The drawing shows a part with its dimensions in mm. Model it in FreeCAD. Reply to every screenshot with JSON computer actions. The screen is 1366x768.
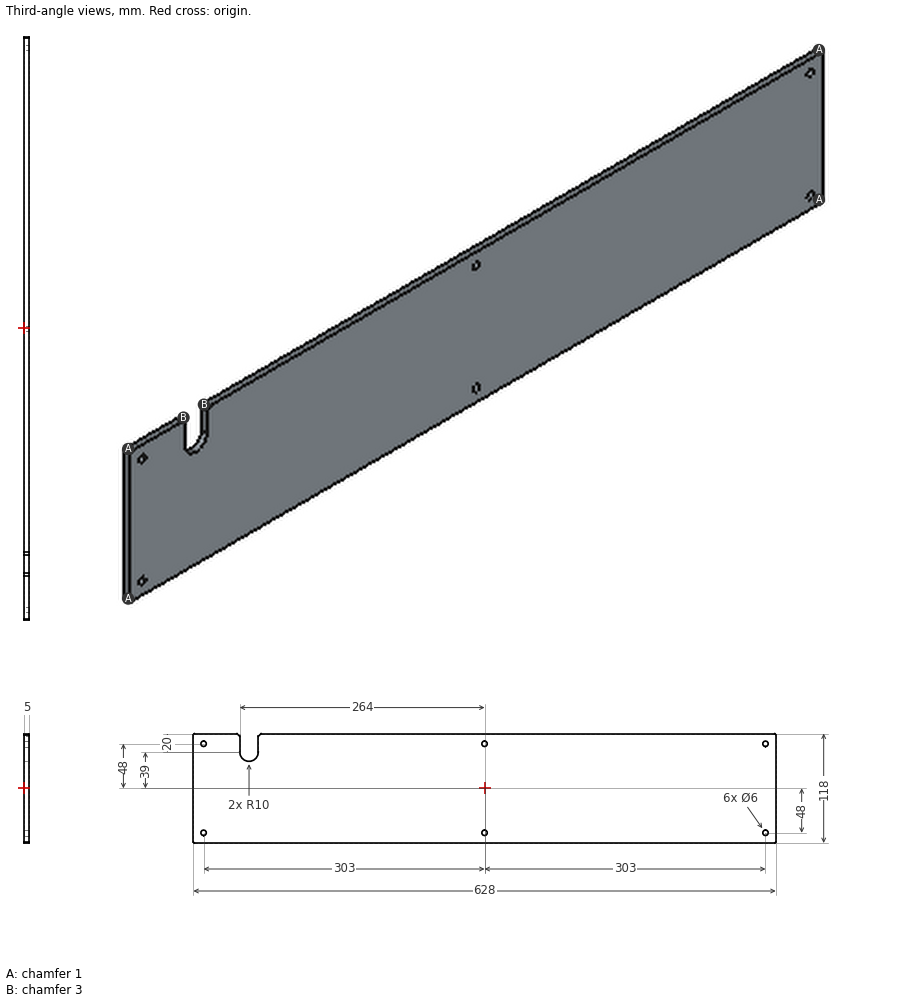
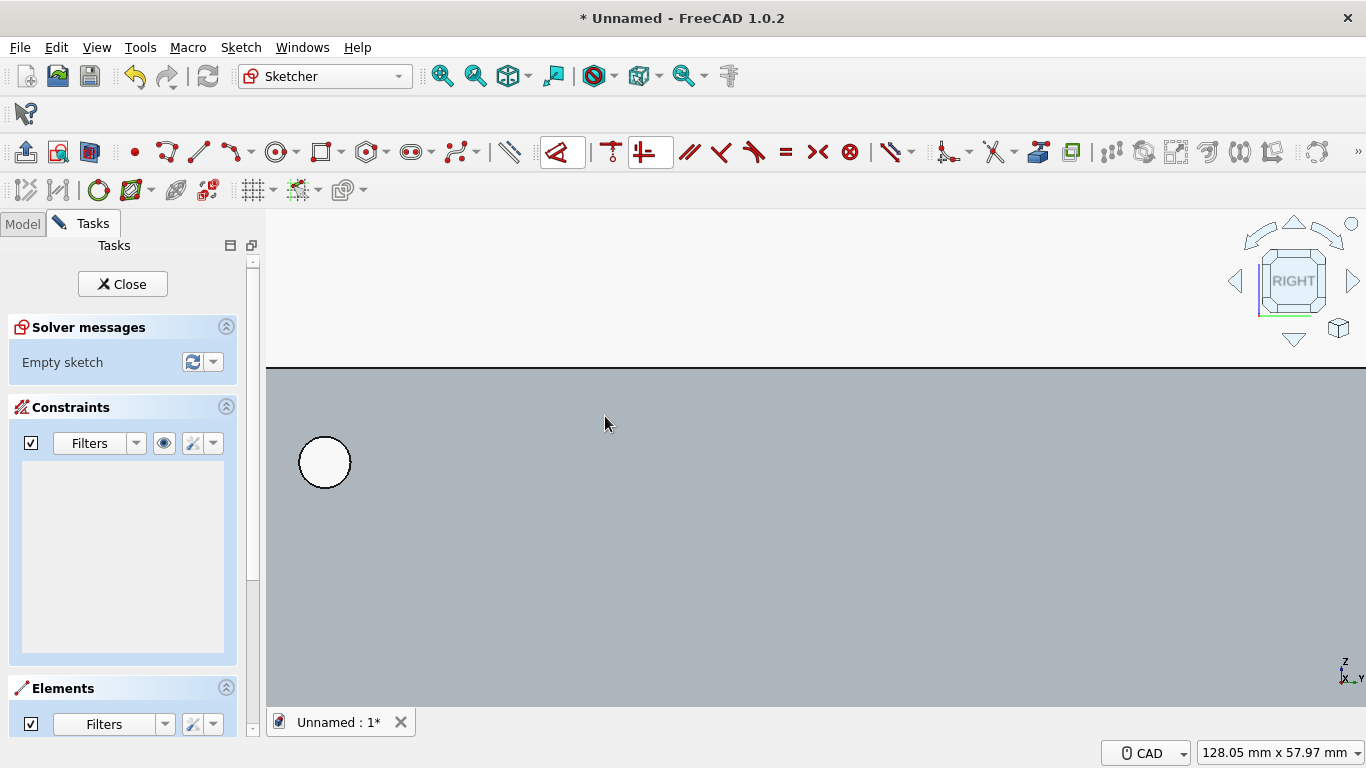
{"action": "left_click", "coordinate": [412, 152]}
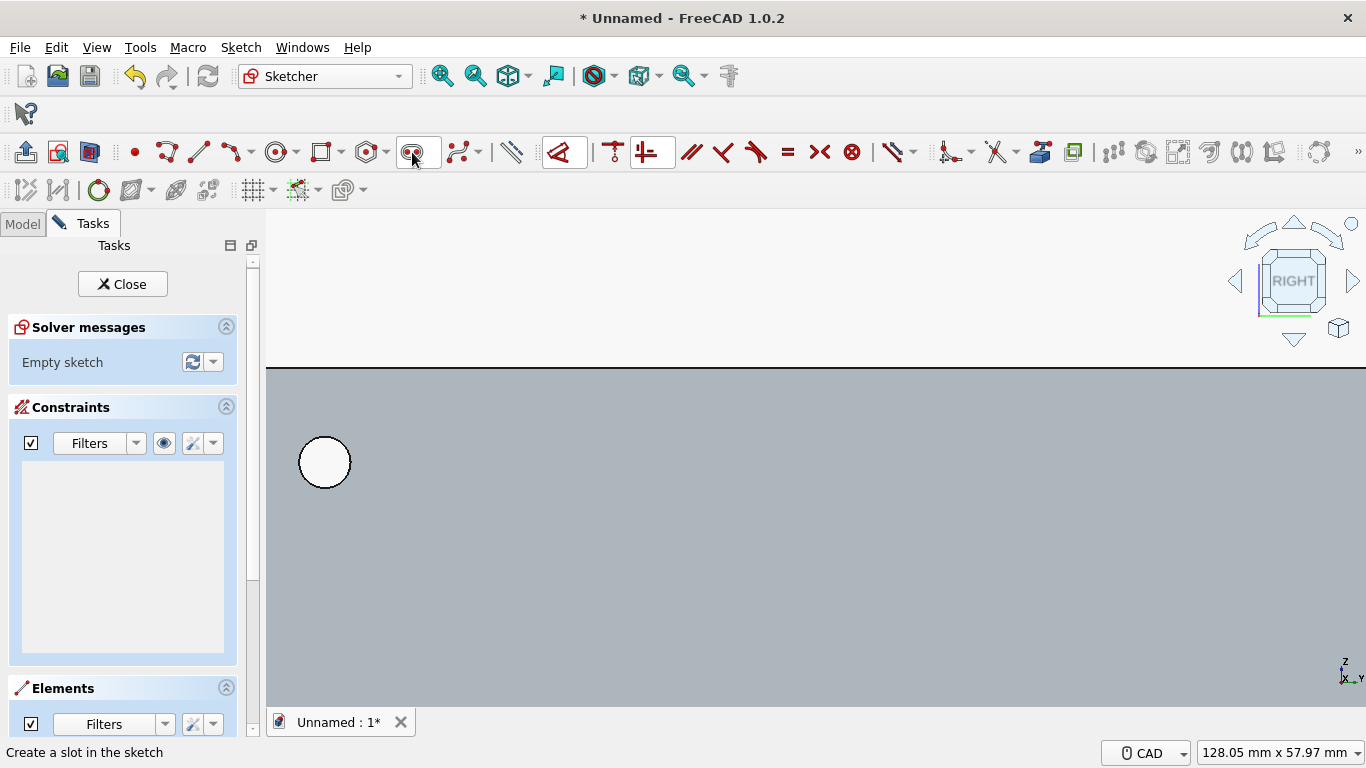
{"action": "left_click", "coordinate": [746, 540]}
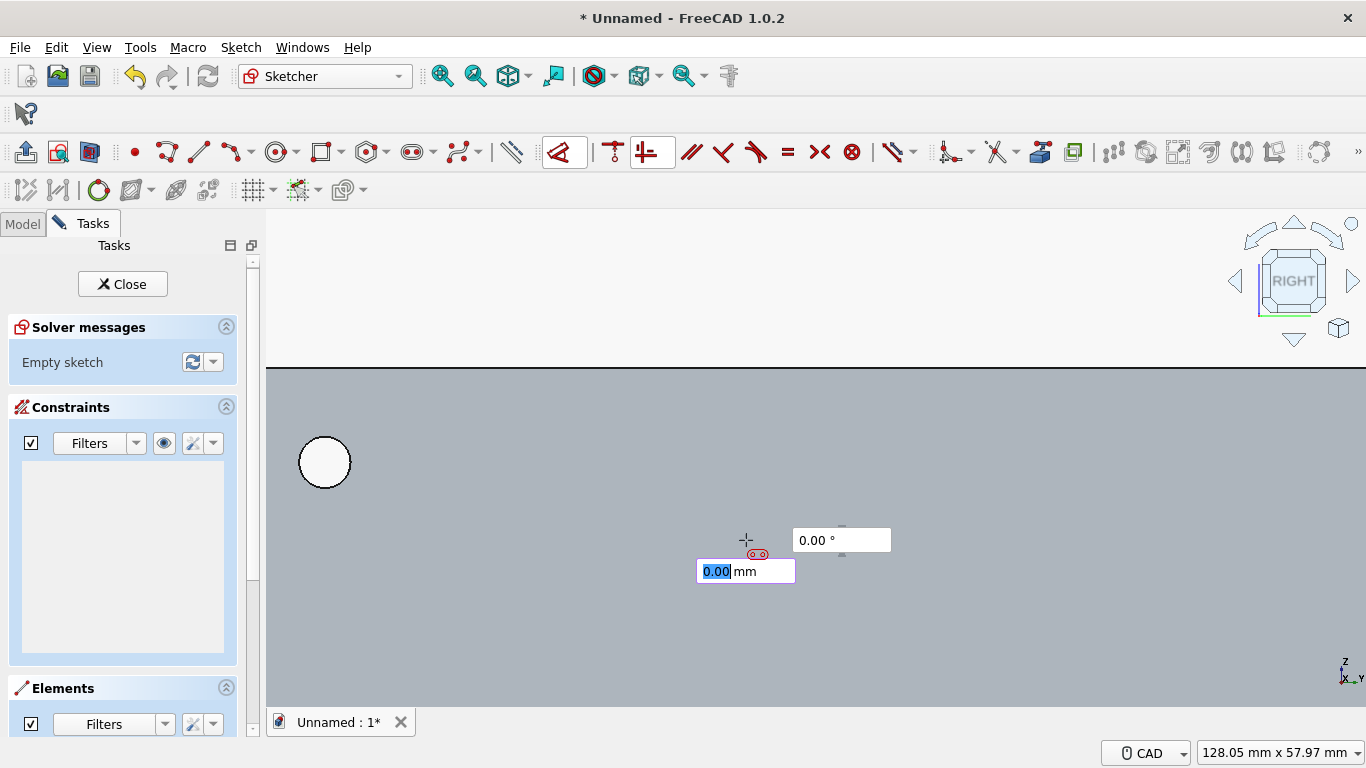
{"action": "left_click", "coordinate": [746, 368]}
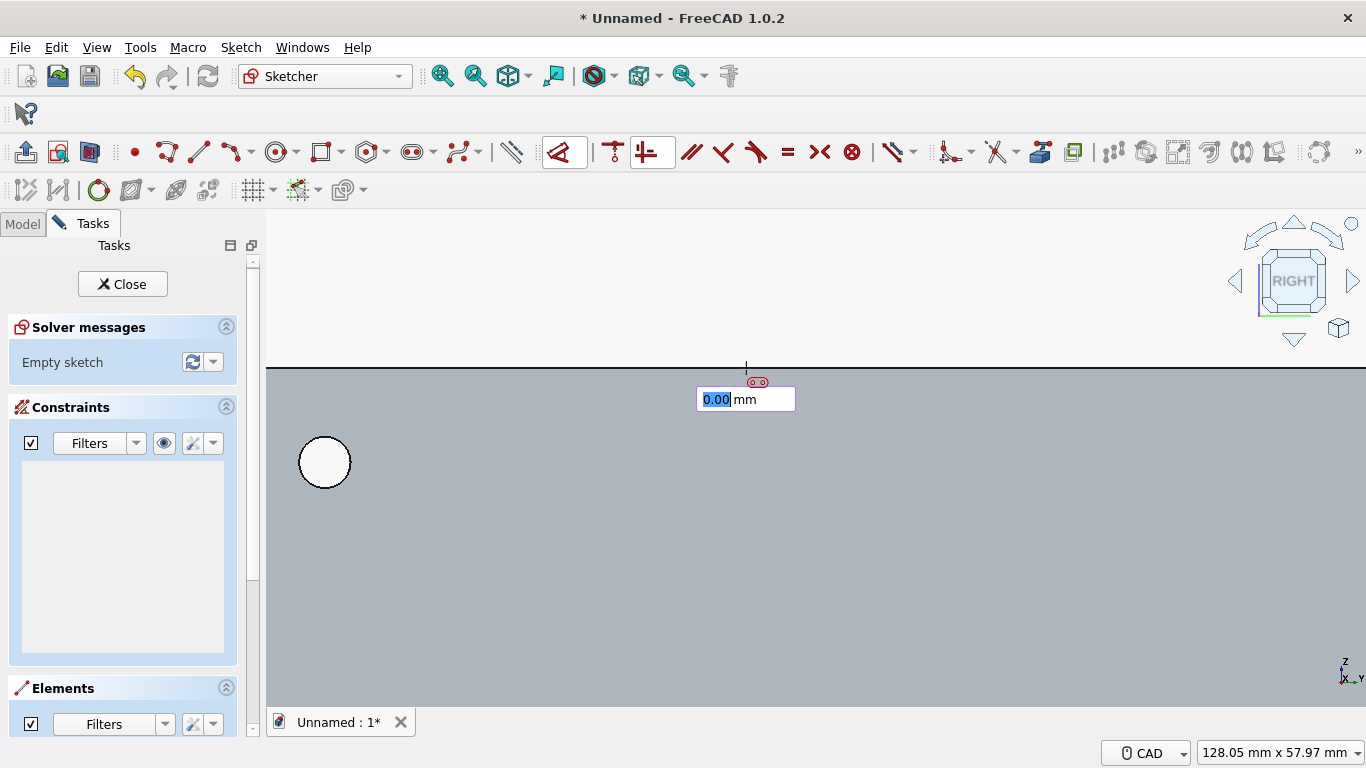
{"action": "left_click", "coordinate": [660, 454]}
{"action": "key", "text": "Escape"}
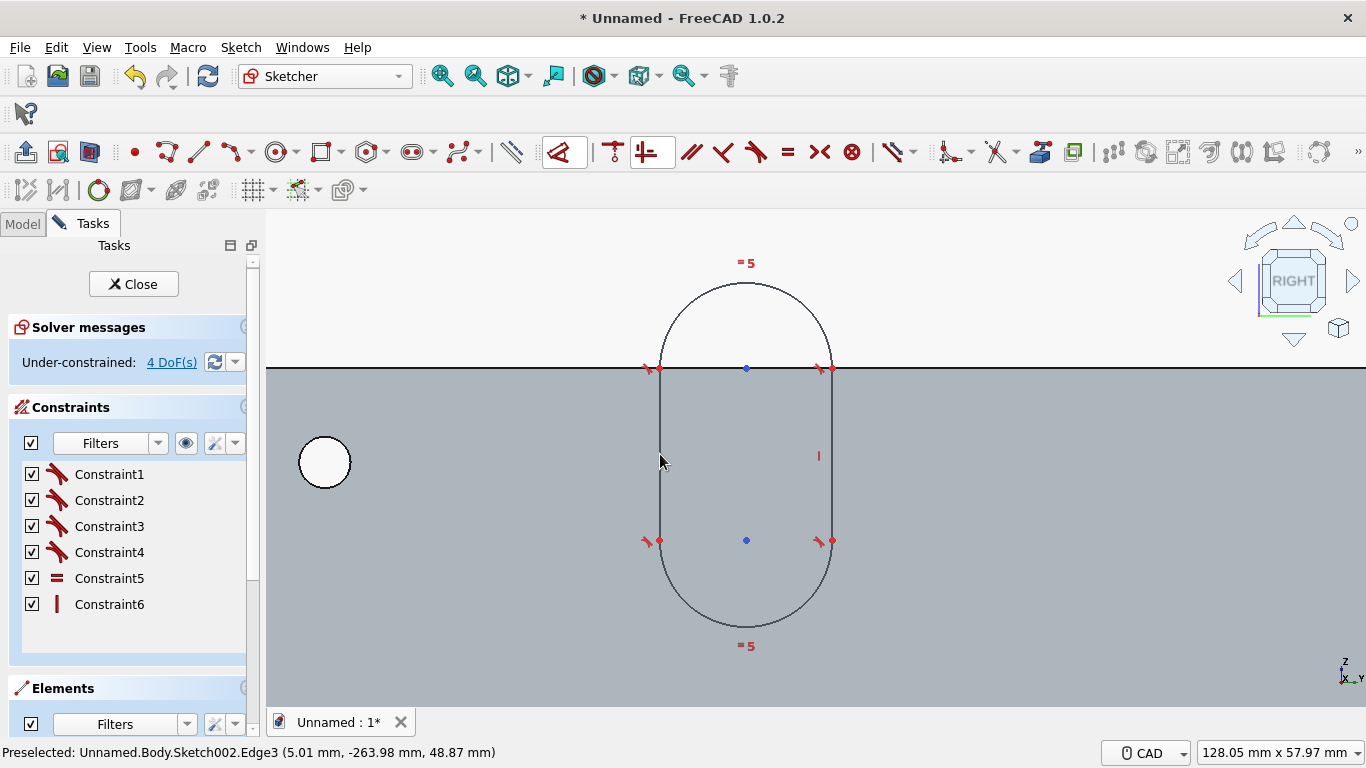
{"action": "left_click", "coordinate": [695, 611]}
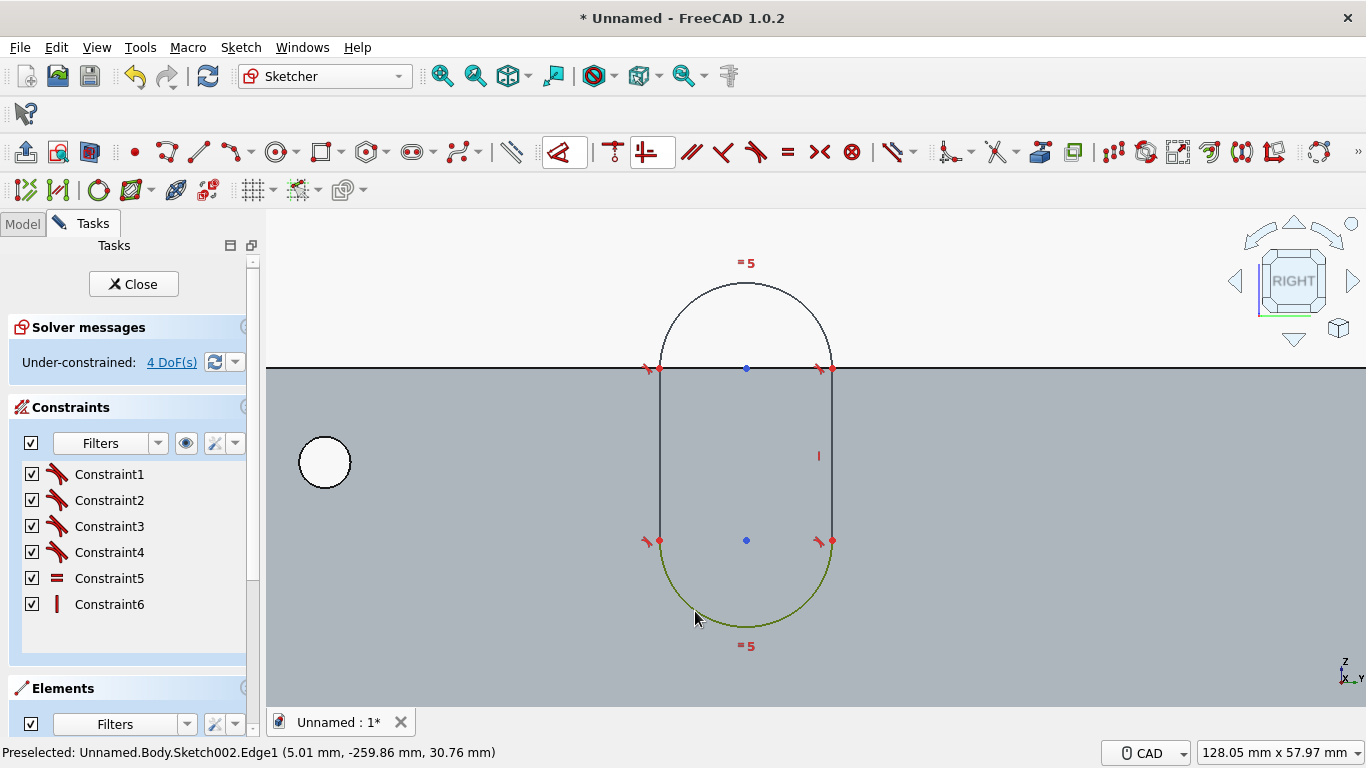
{"action": "key", "text": "k r"}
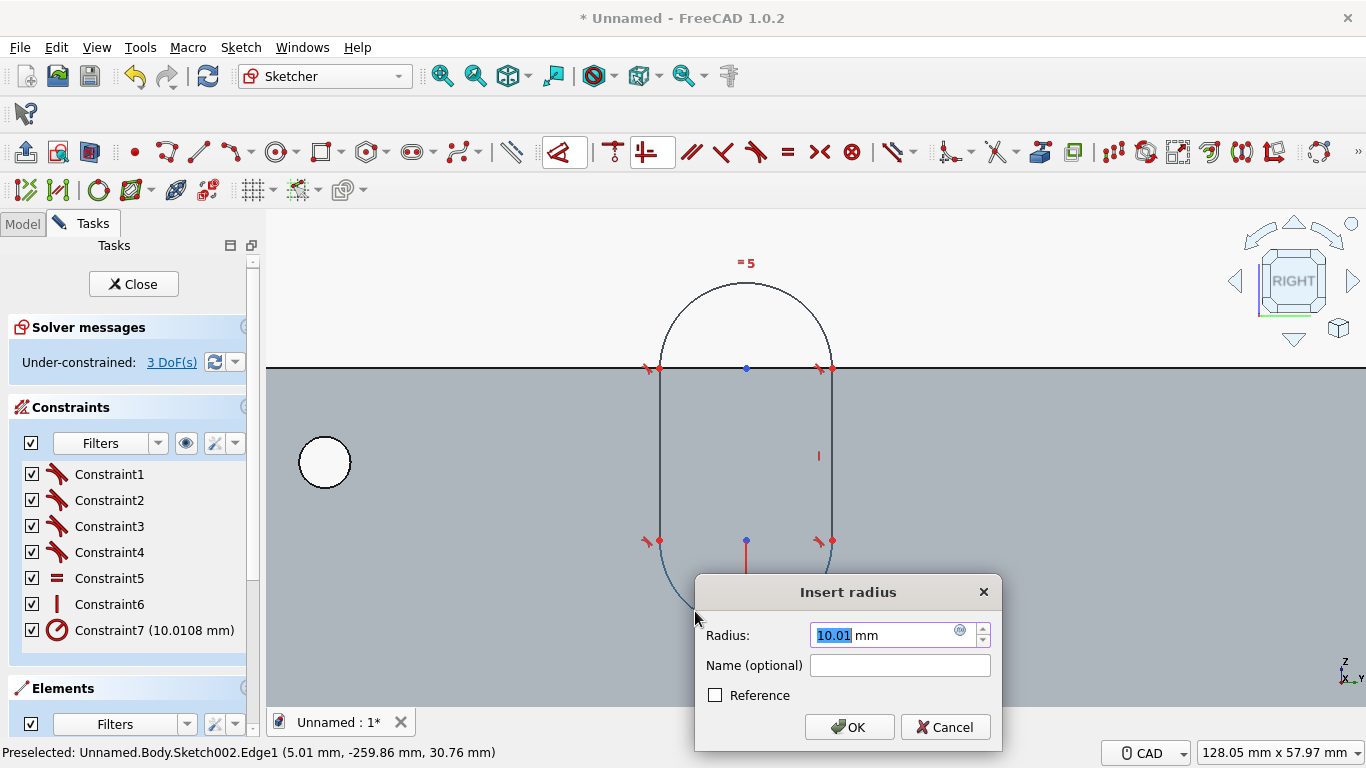
{"action": "type", "text": "10"}
{"action": "key", "text": "Return"}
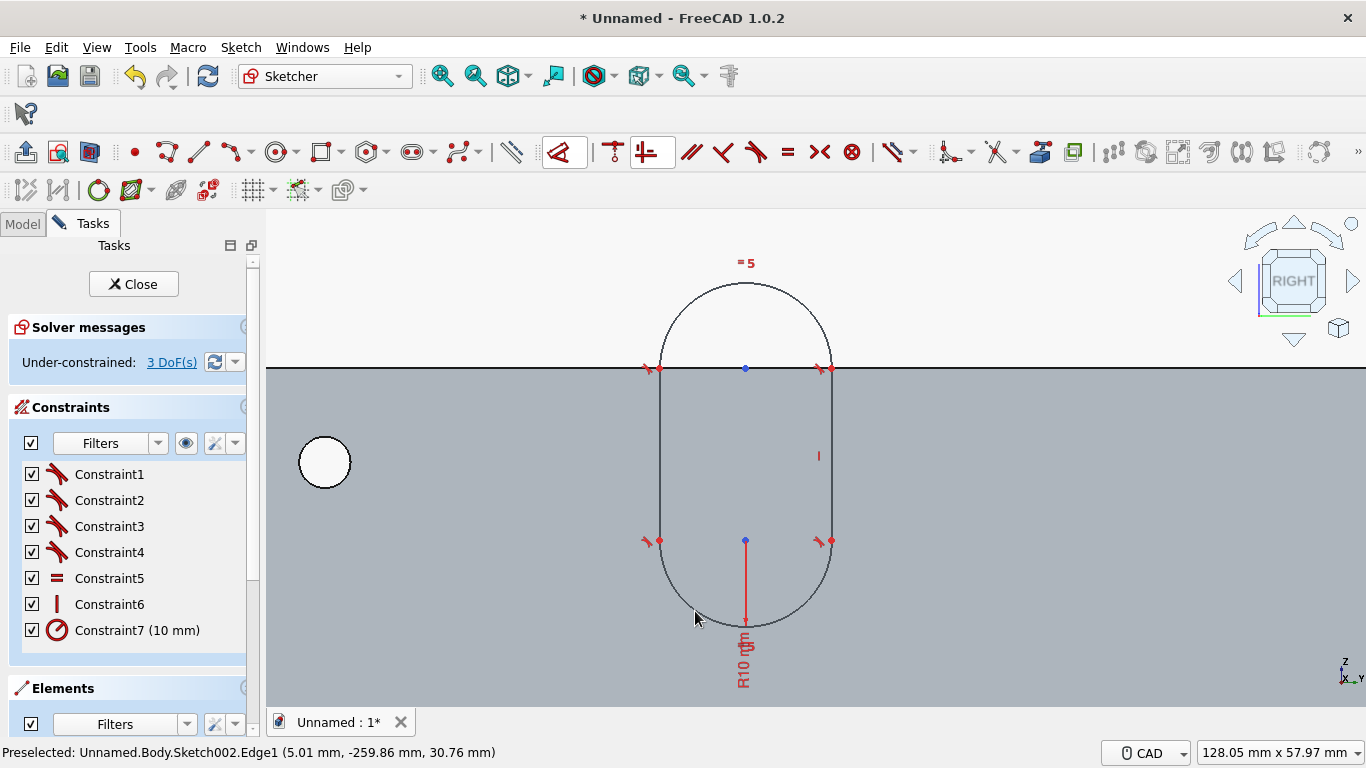
{"action": "left_click", "coordinate": [660, 489]}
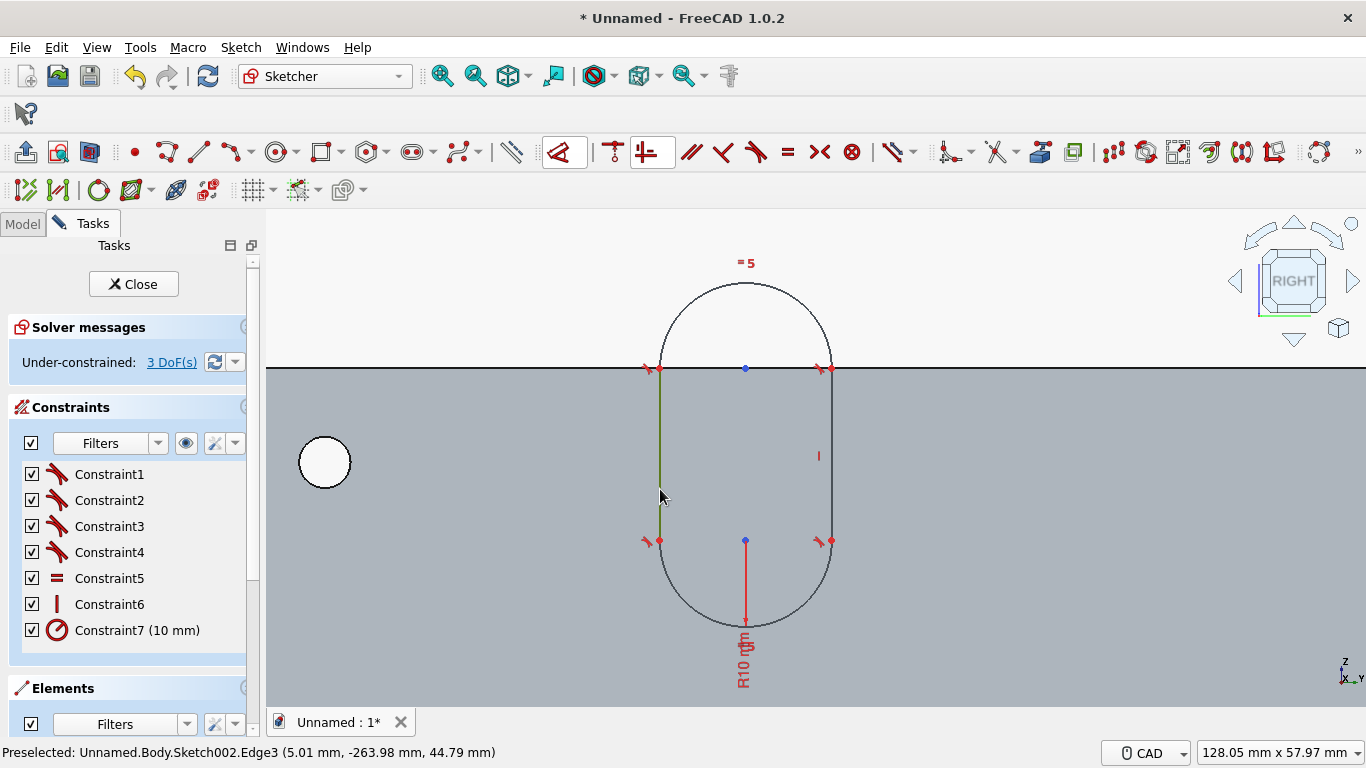
{"action": "left_click", "coordinate": [582, 152]}